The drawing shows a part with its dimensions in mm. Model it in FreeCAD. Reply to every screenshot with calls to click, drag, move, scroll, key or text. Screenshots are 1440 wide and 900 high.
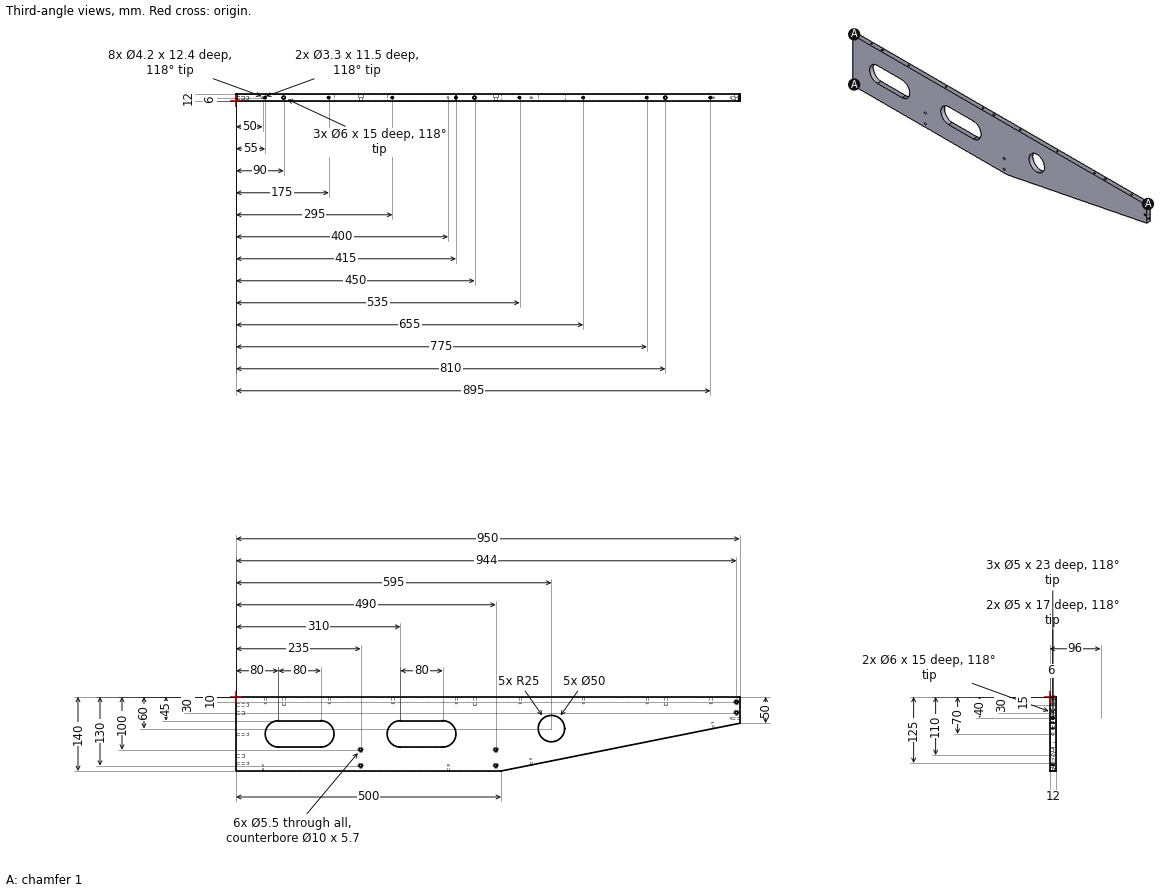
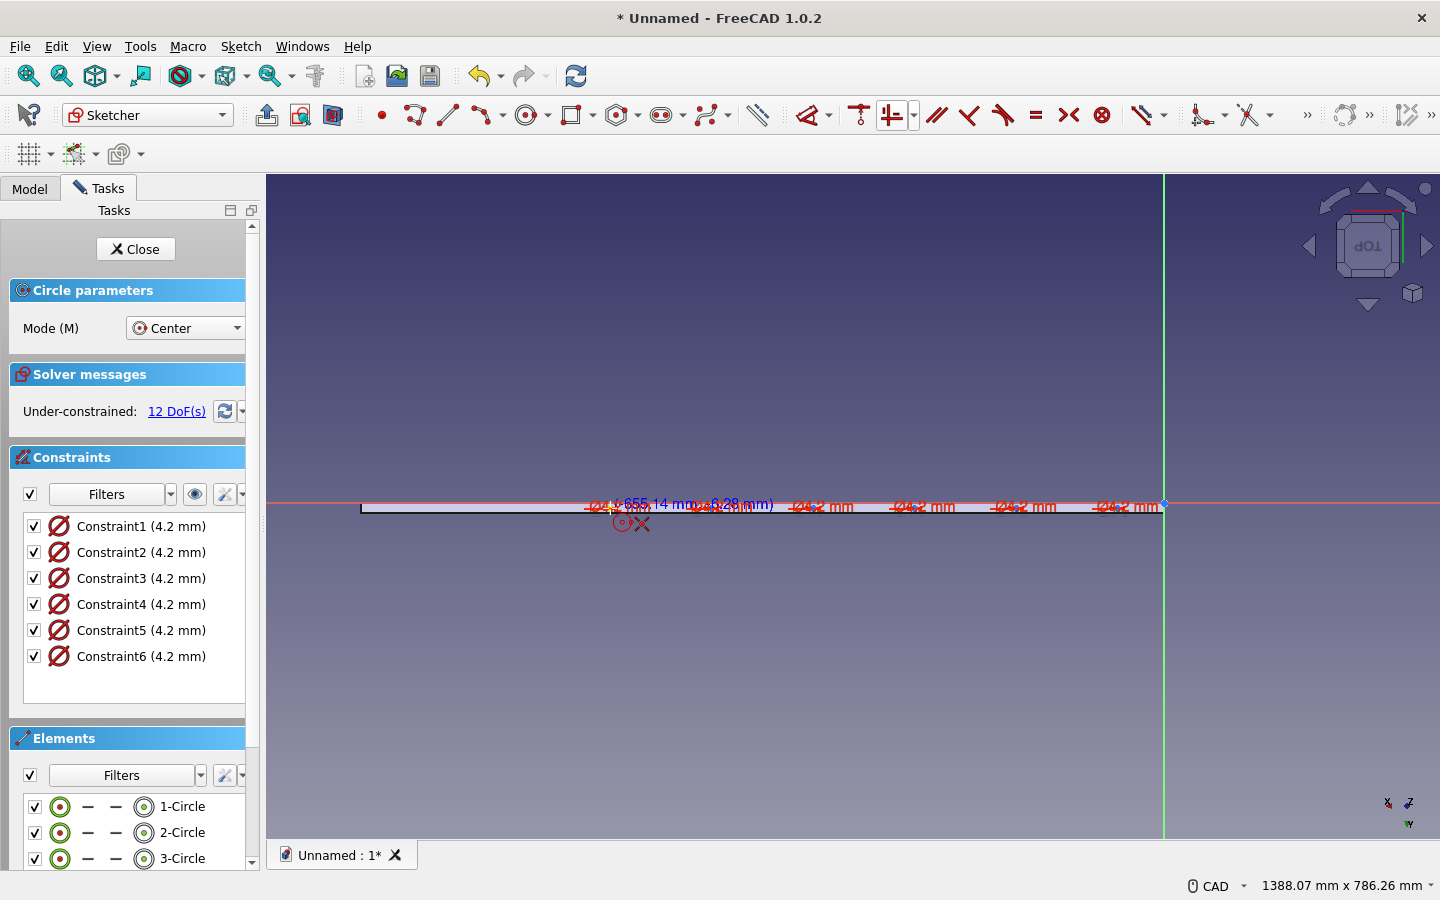
scroll(509, 508, up, 13)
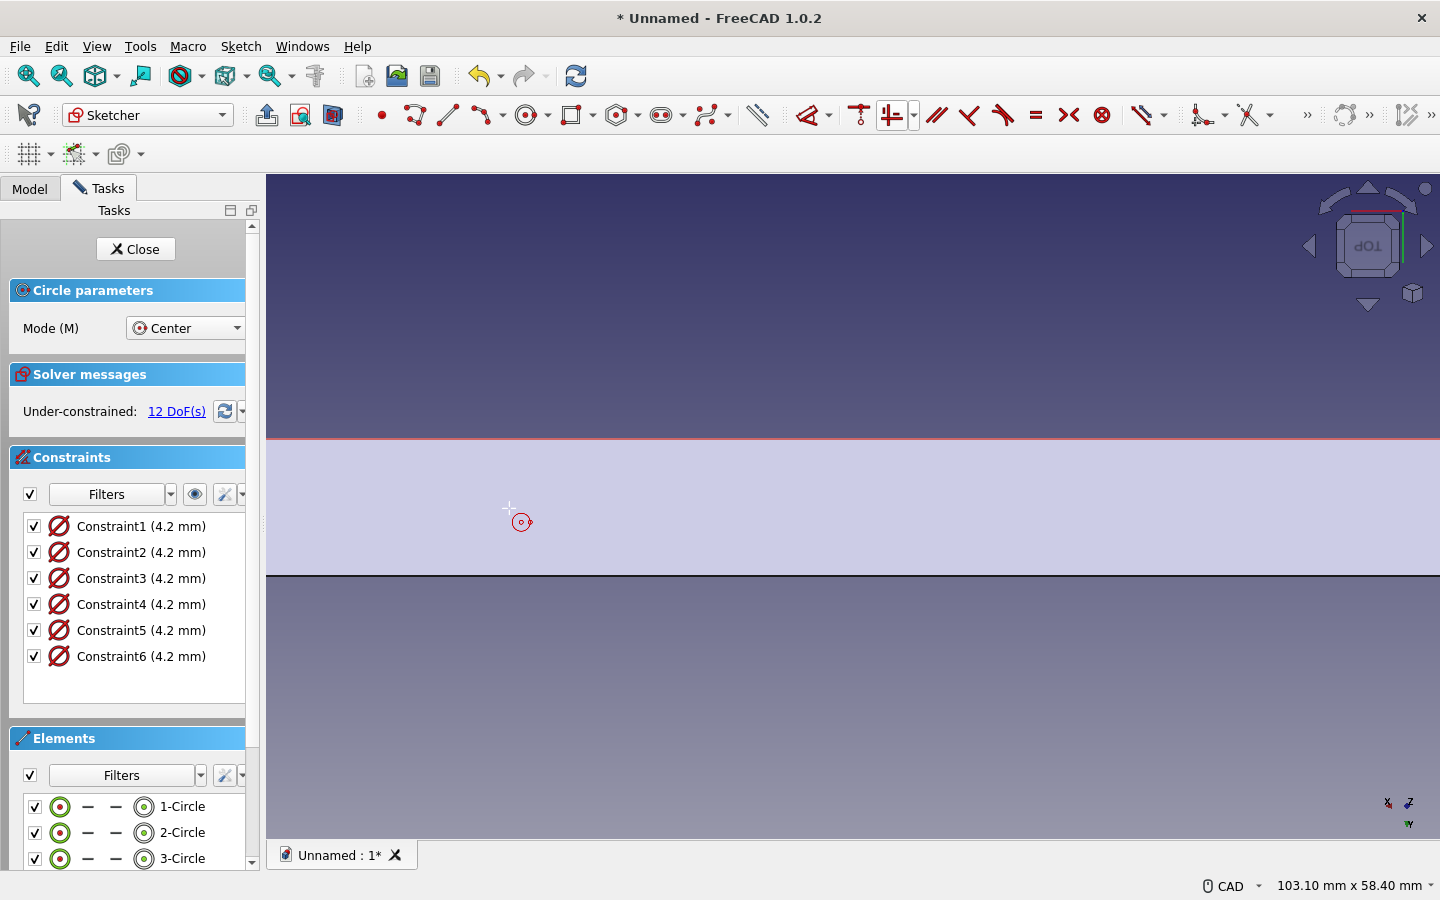
scroll(509, 508, down, 13)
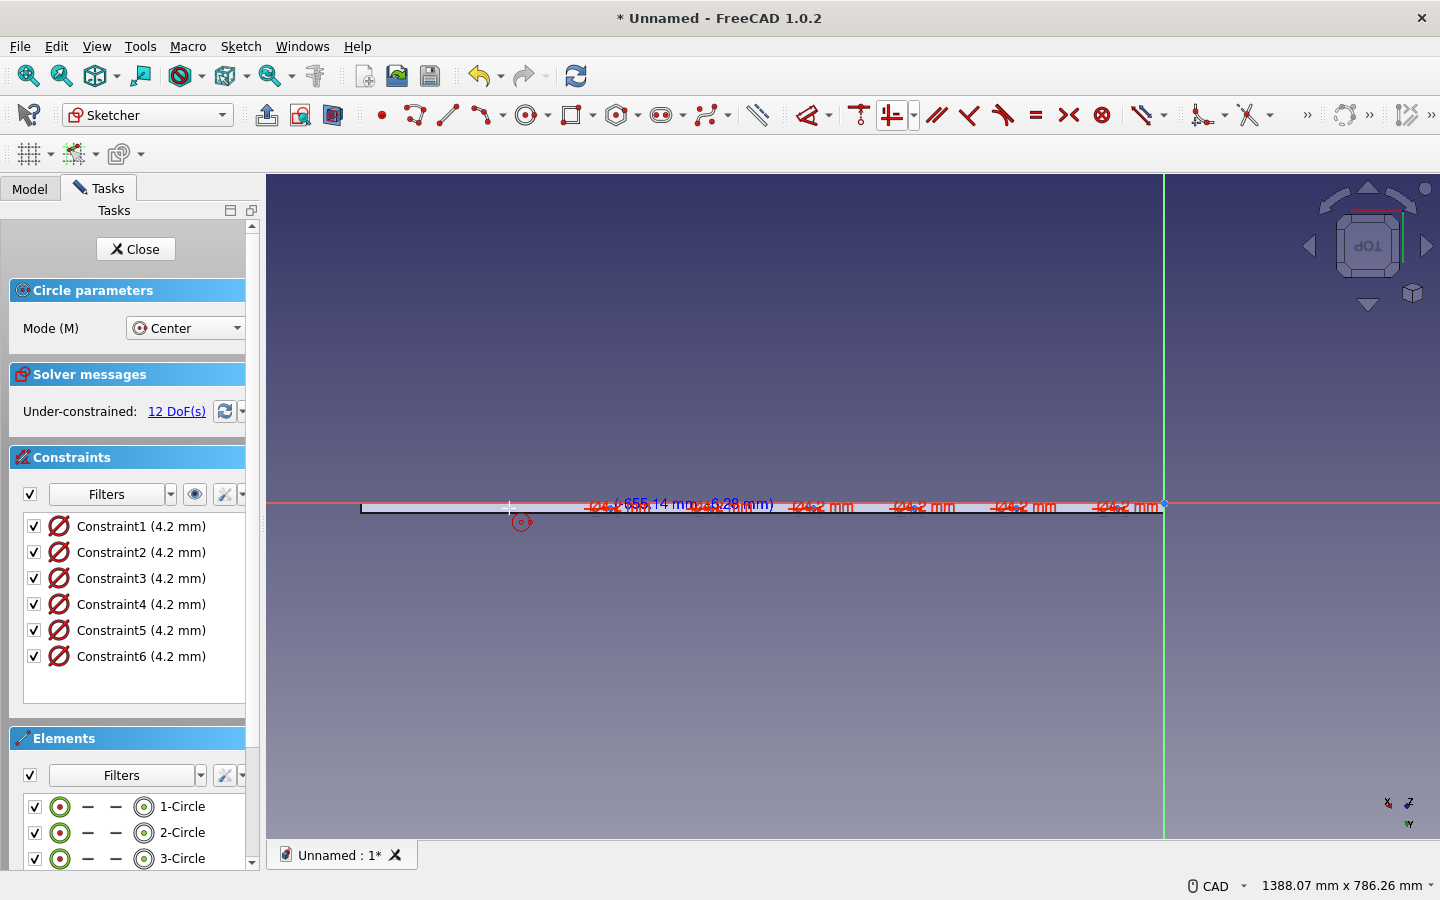
scroll(509, 508, up, 6)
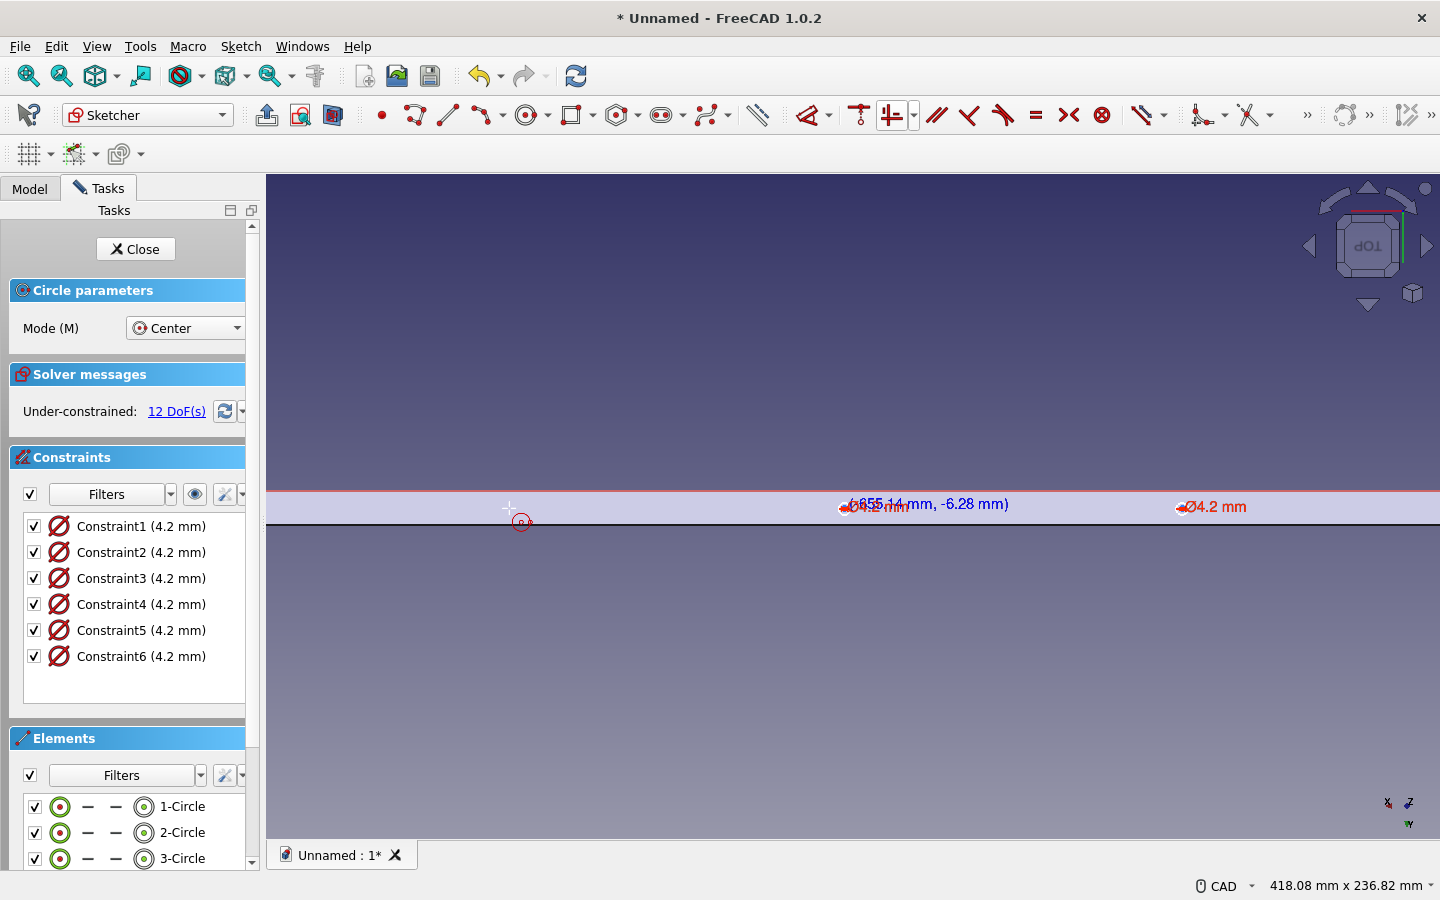
click(508, 508)
move(512, 512)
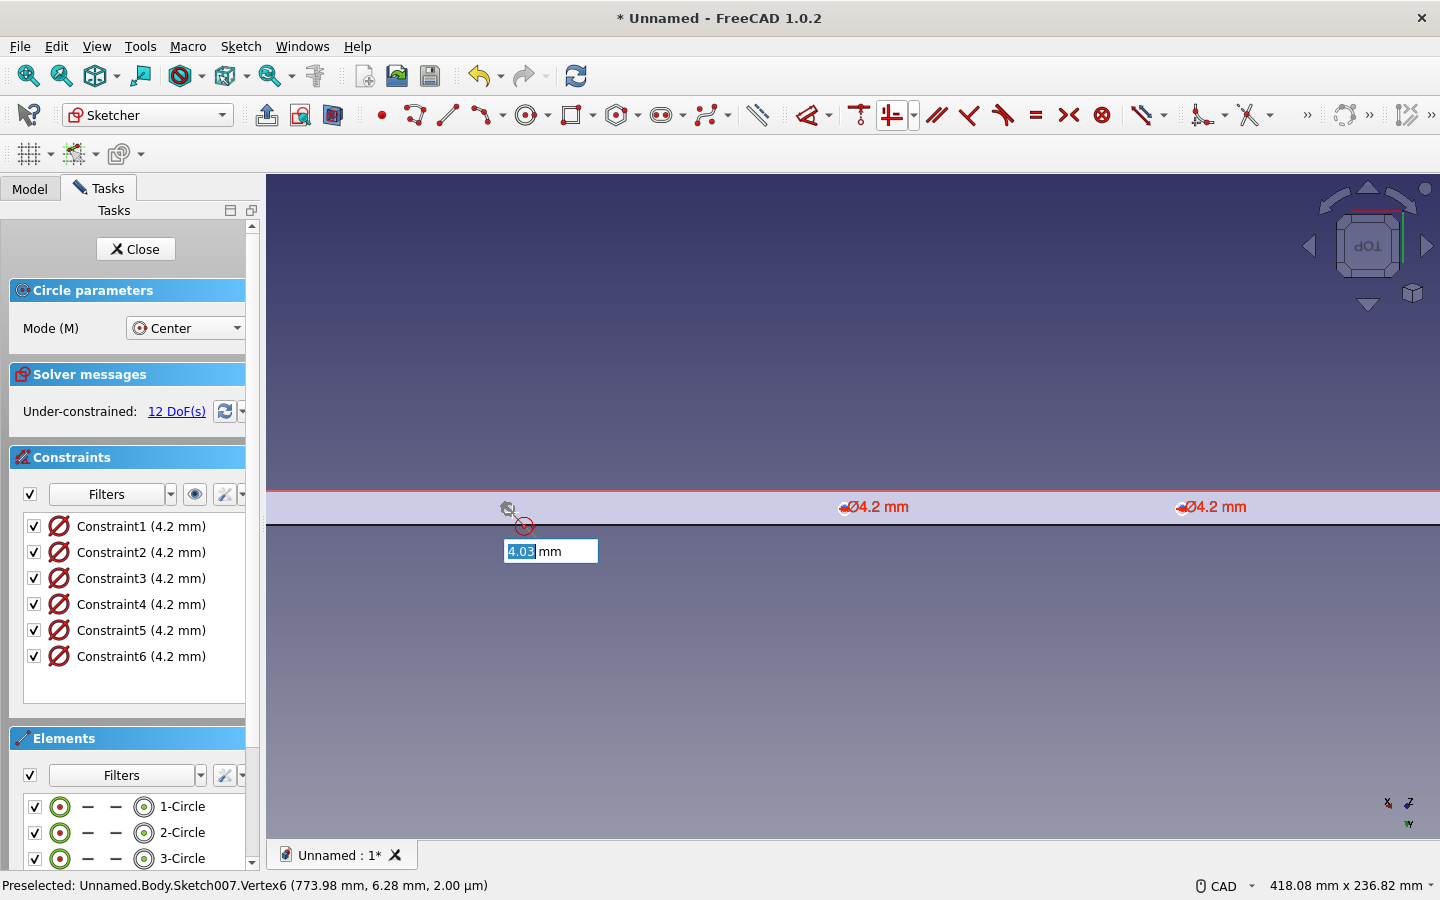
text(4.2)
key(Return)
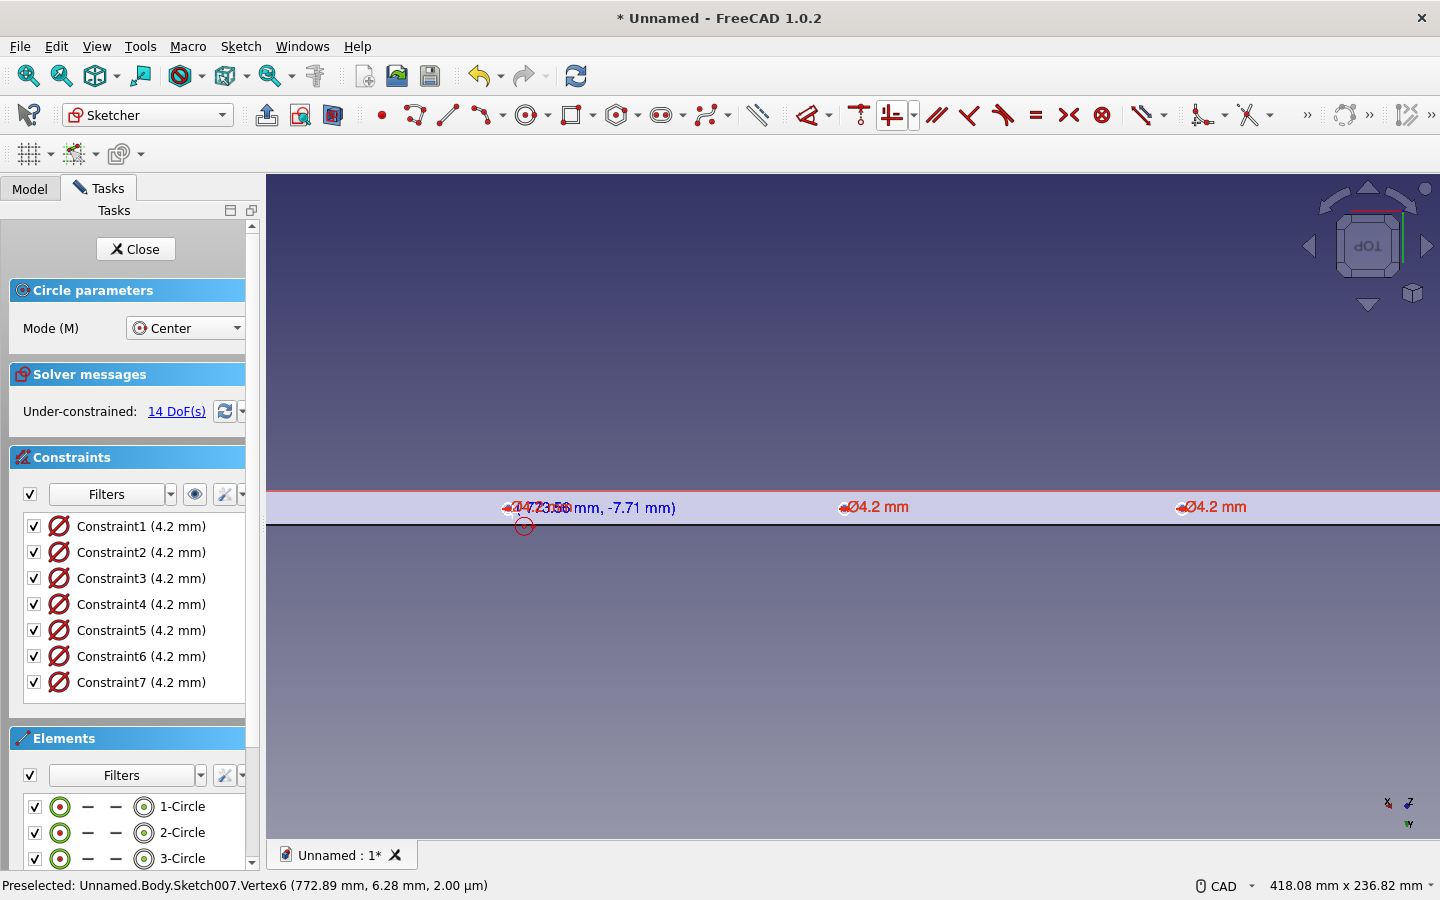
scroll(509, 508, down, 6)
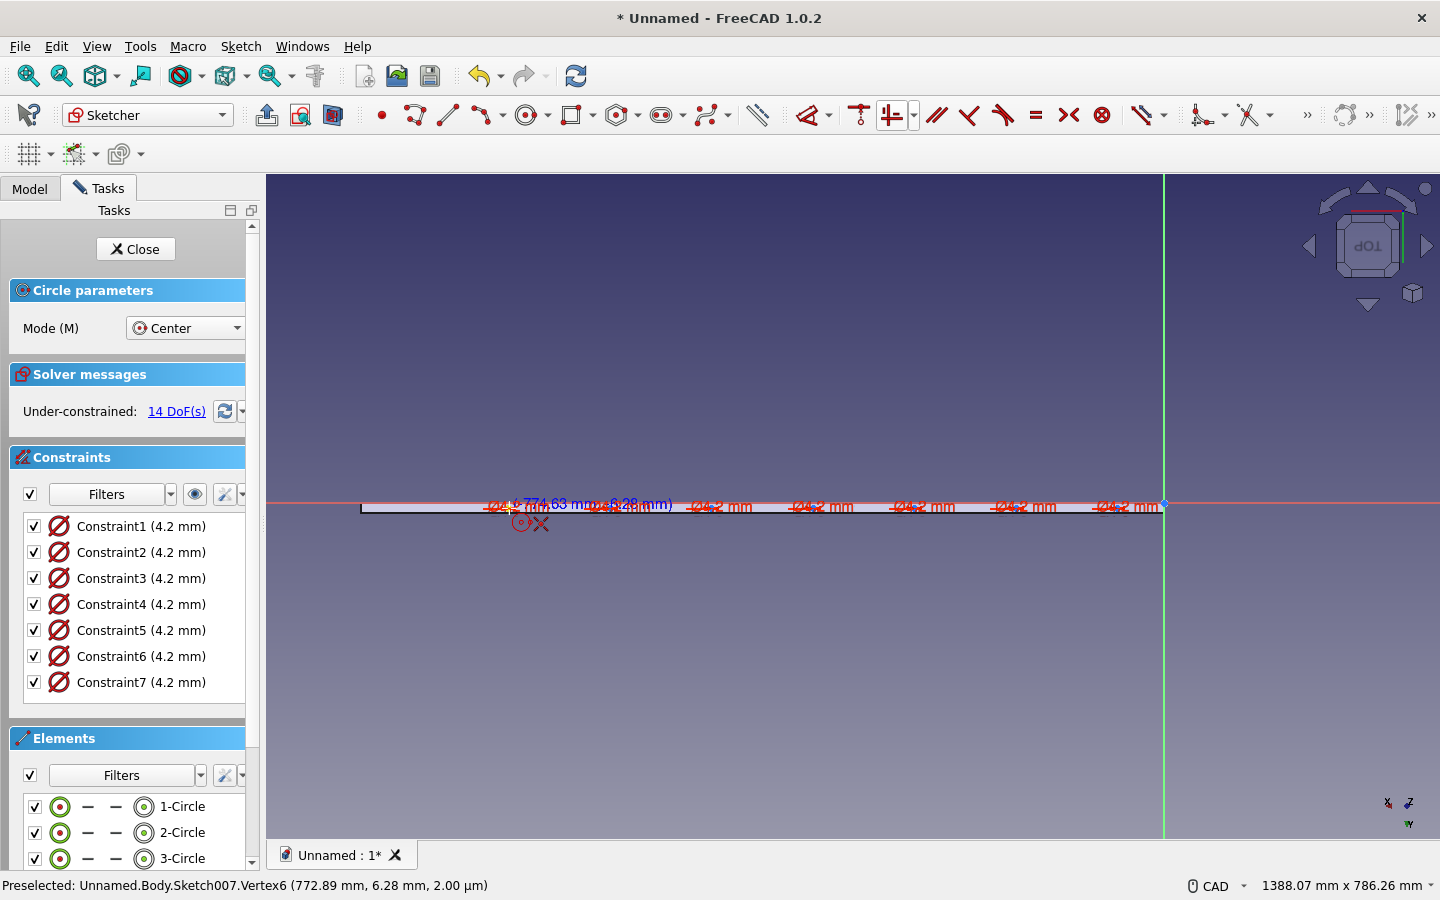
scroll(407, 508, up, 13)